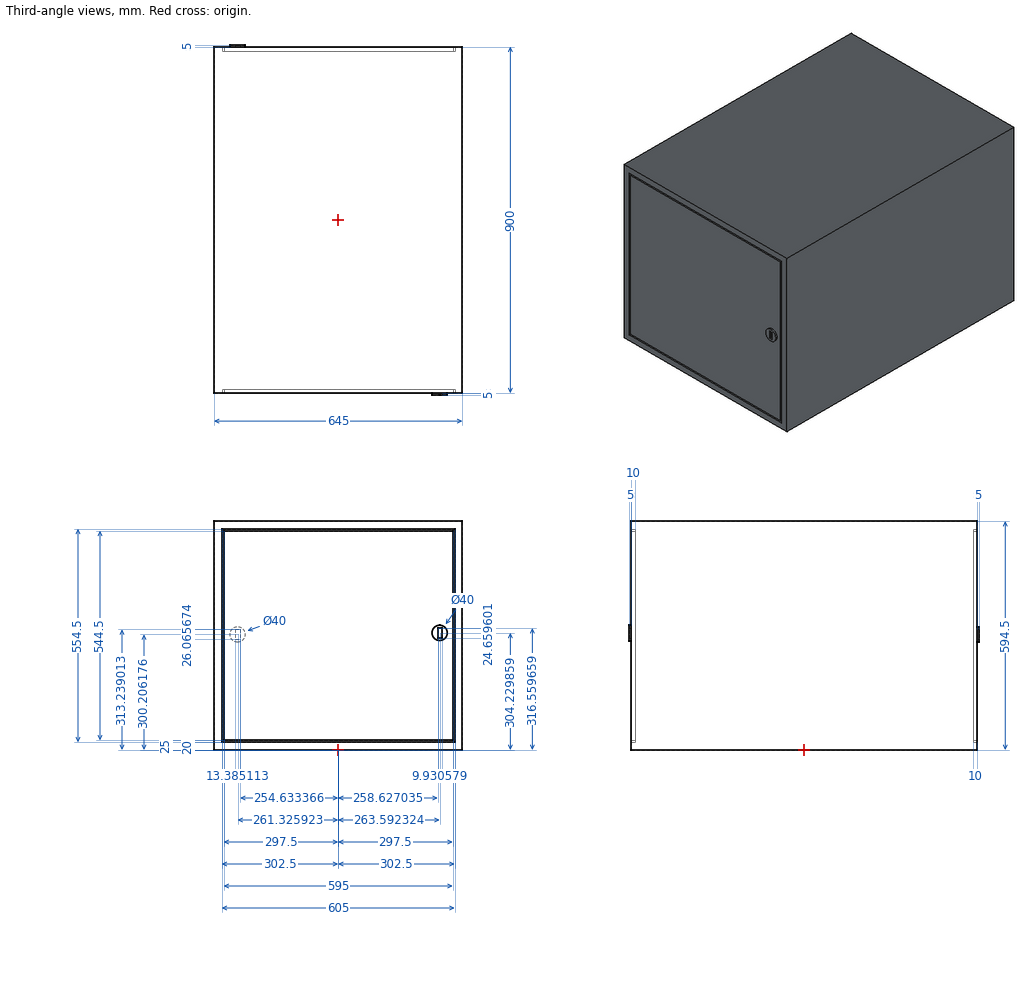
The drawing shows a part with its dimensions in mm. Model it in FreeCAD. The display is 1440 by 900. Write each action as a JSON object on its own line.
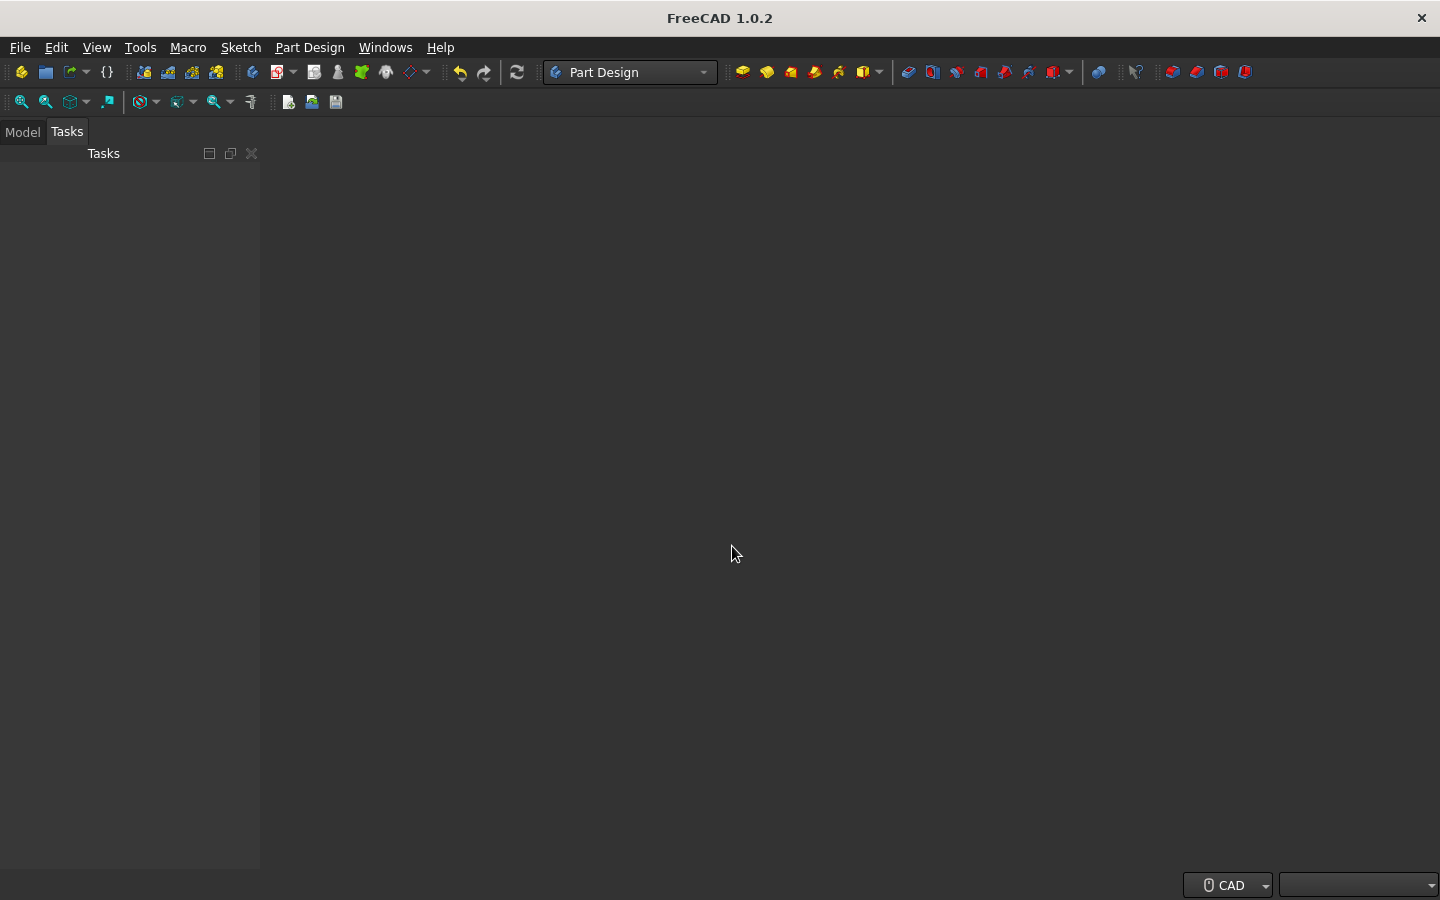
{"action": "key", "text": "ctrl+n"}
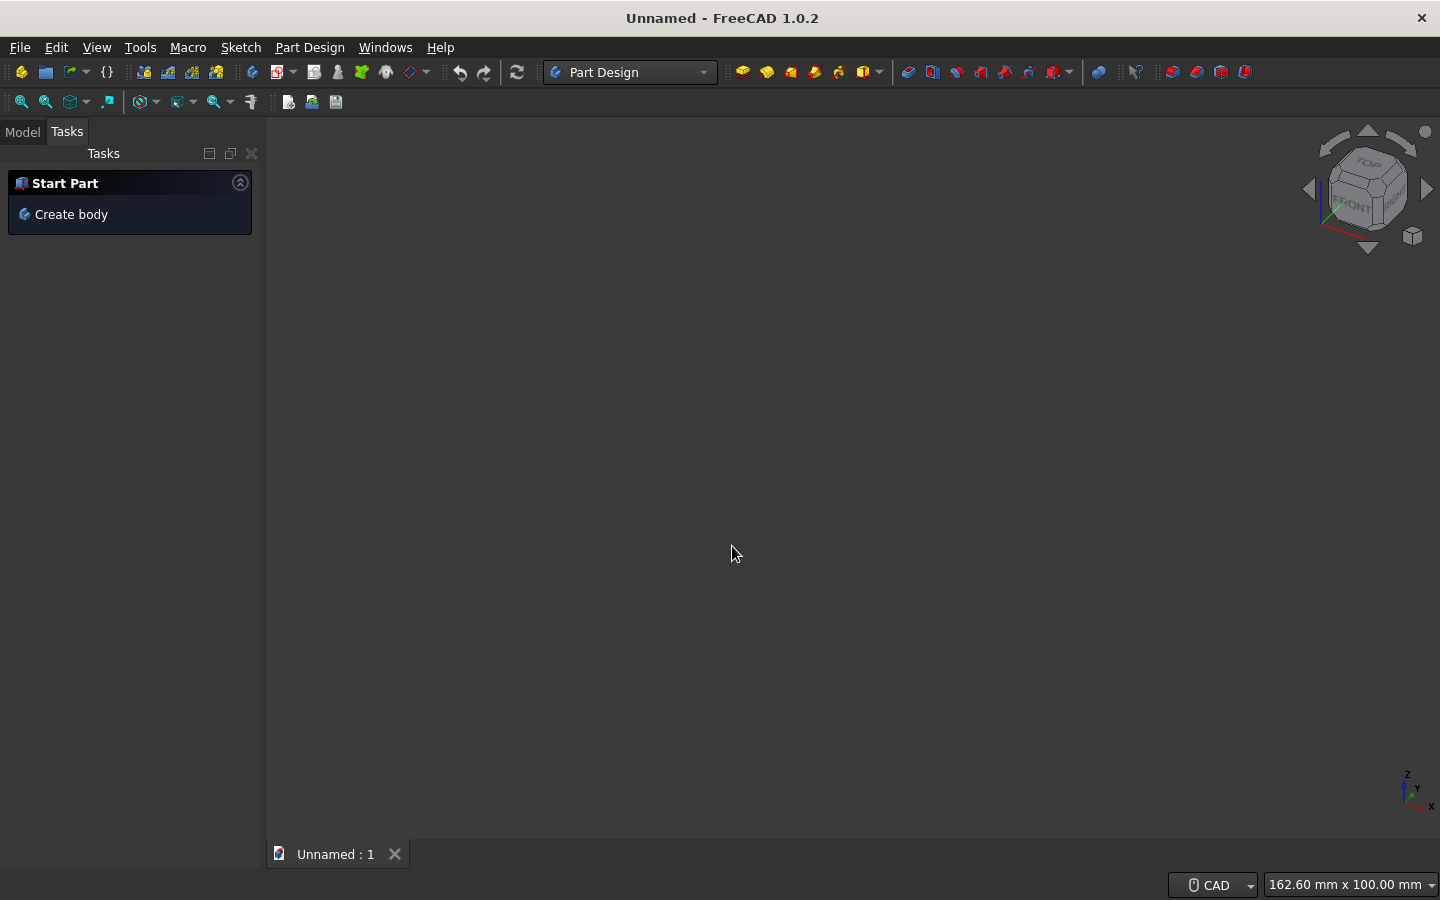
{"action": "left_click", "coordinate": [278, 72]}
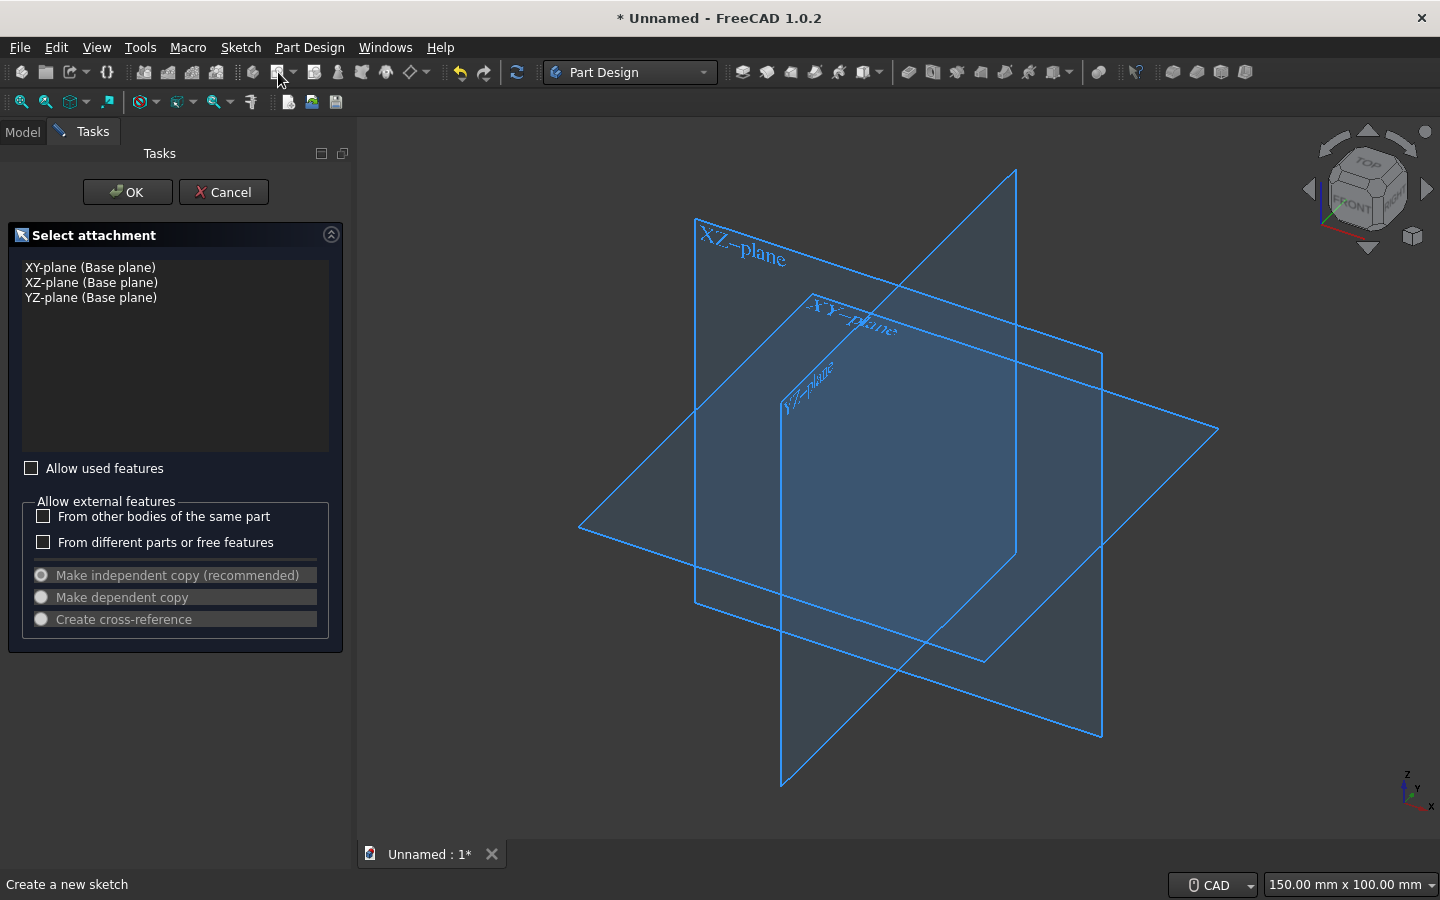
{"action": "left_click", "coordinate": [82, 268]}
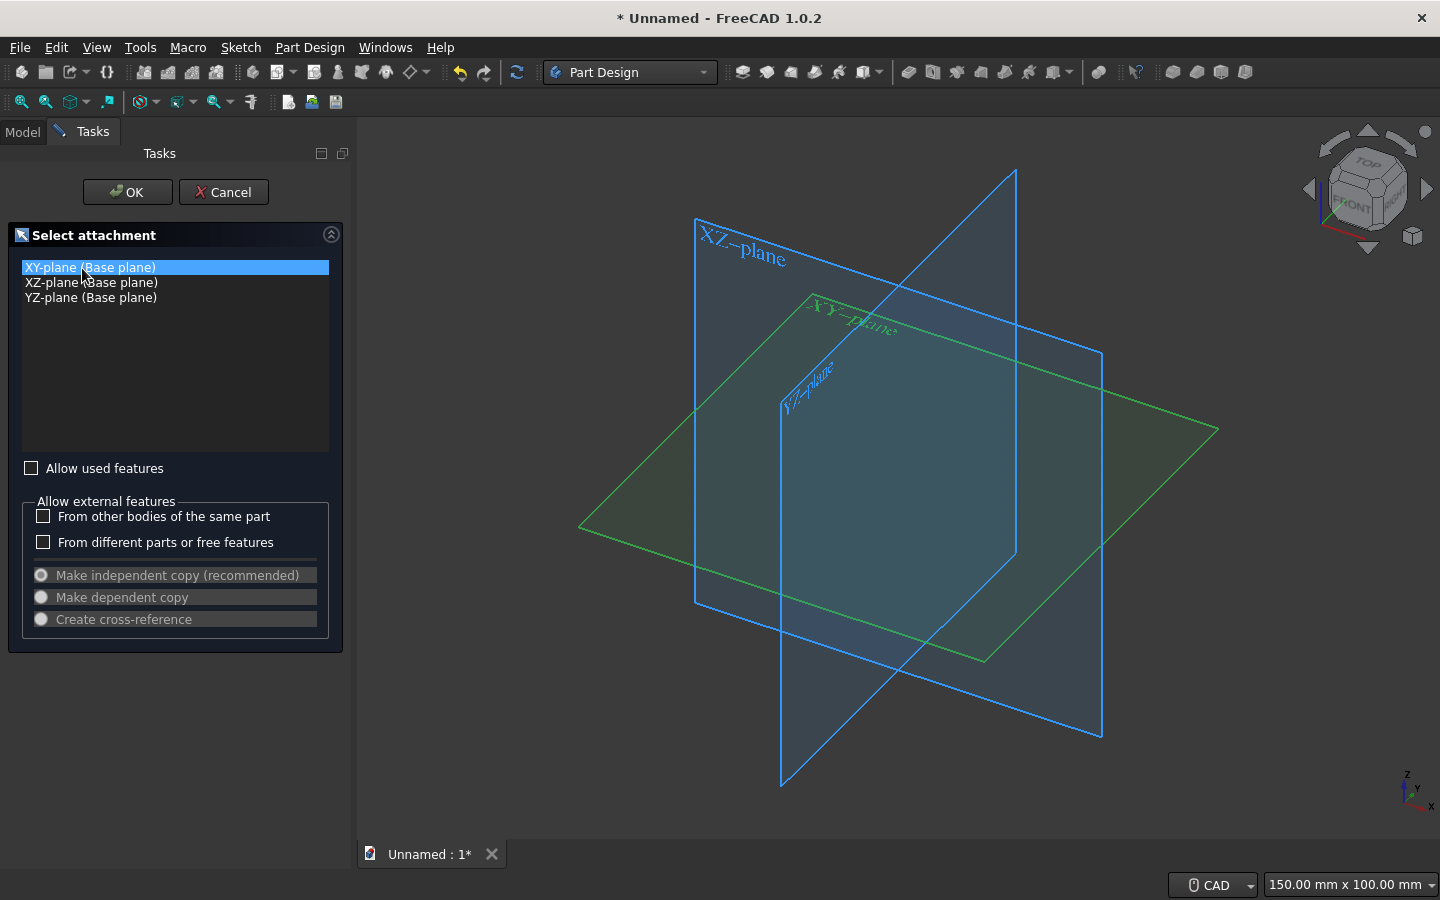
{"action": "left_click", "coordinate": [128, 192]}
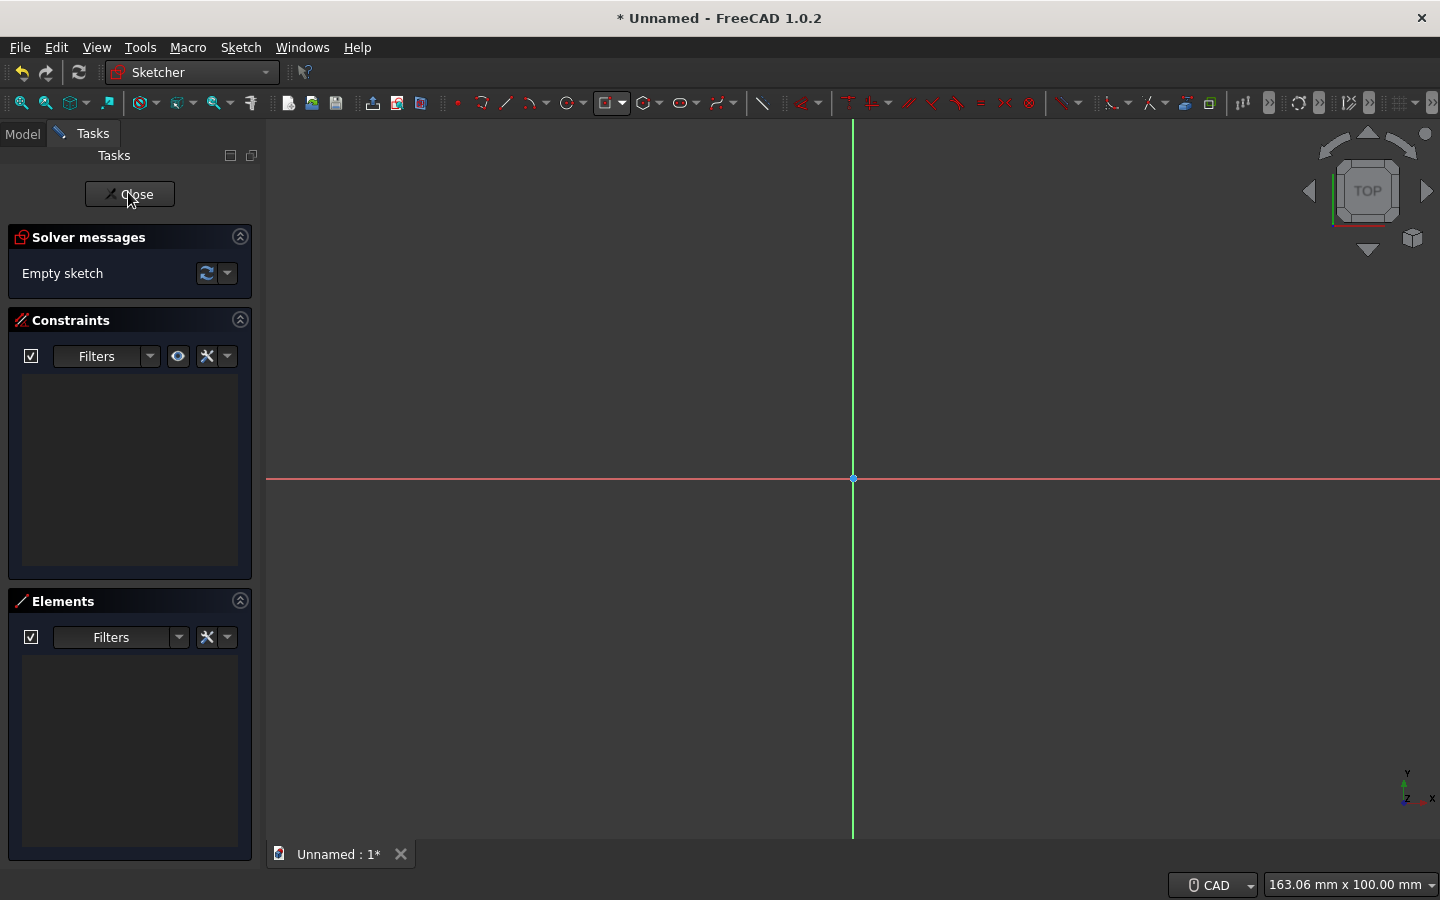
{"action": "scroll", "coordinate": [779, 479], "scroll_direction": "down", "scroll_amount": 13}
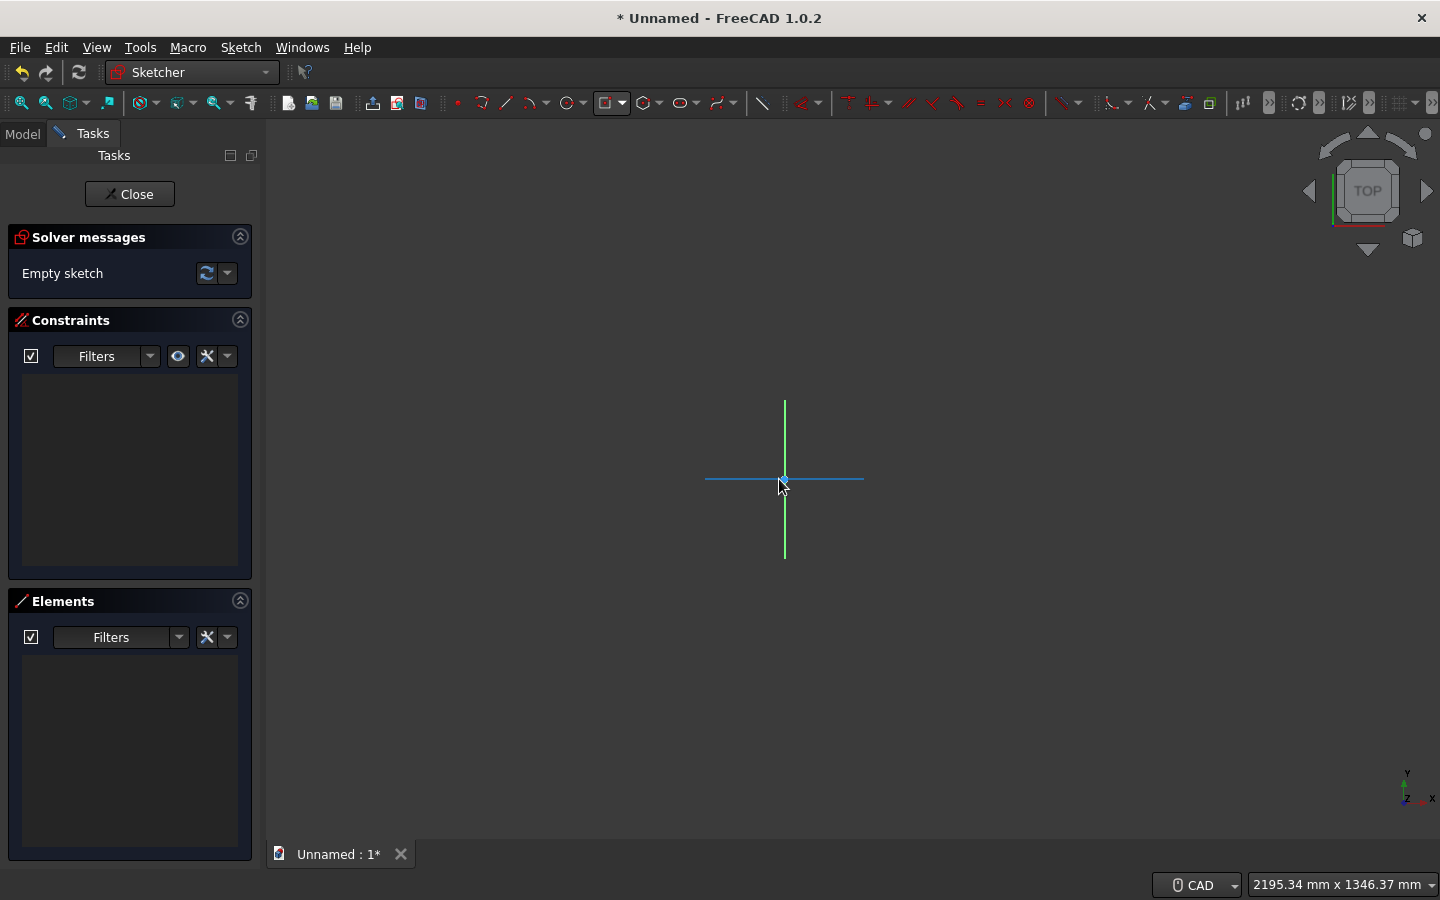
{"action": "key", "text": "g v"}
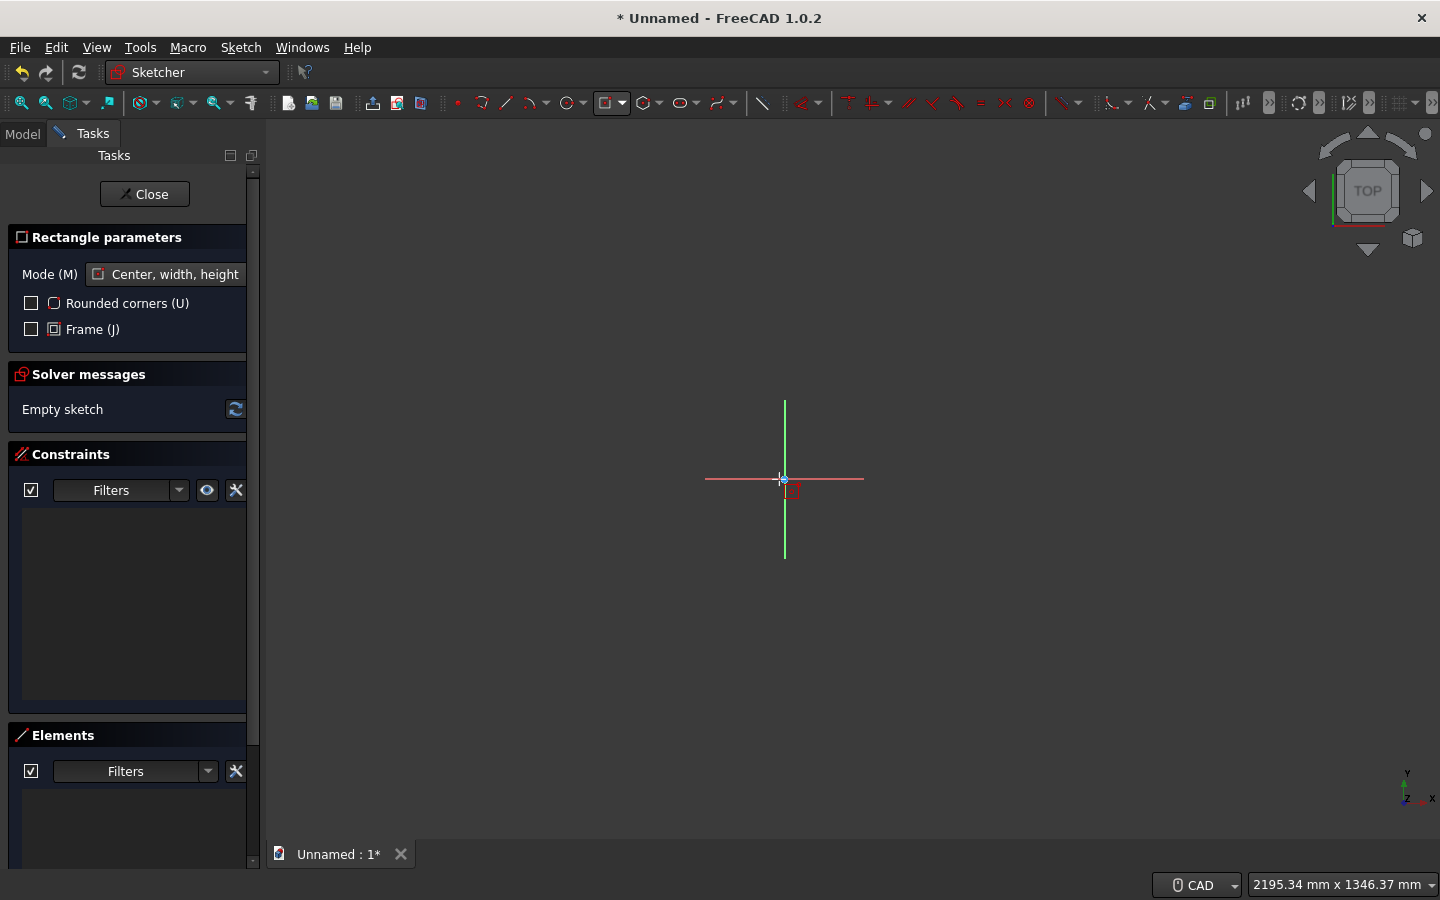
{"action": "left_click", "coordinate": [785, 479]}
{"action": "left_click", "coordinate": [957, 239]}
{"action": "key", "text": "Escape"}